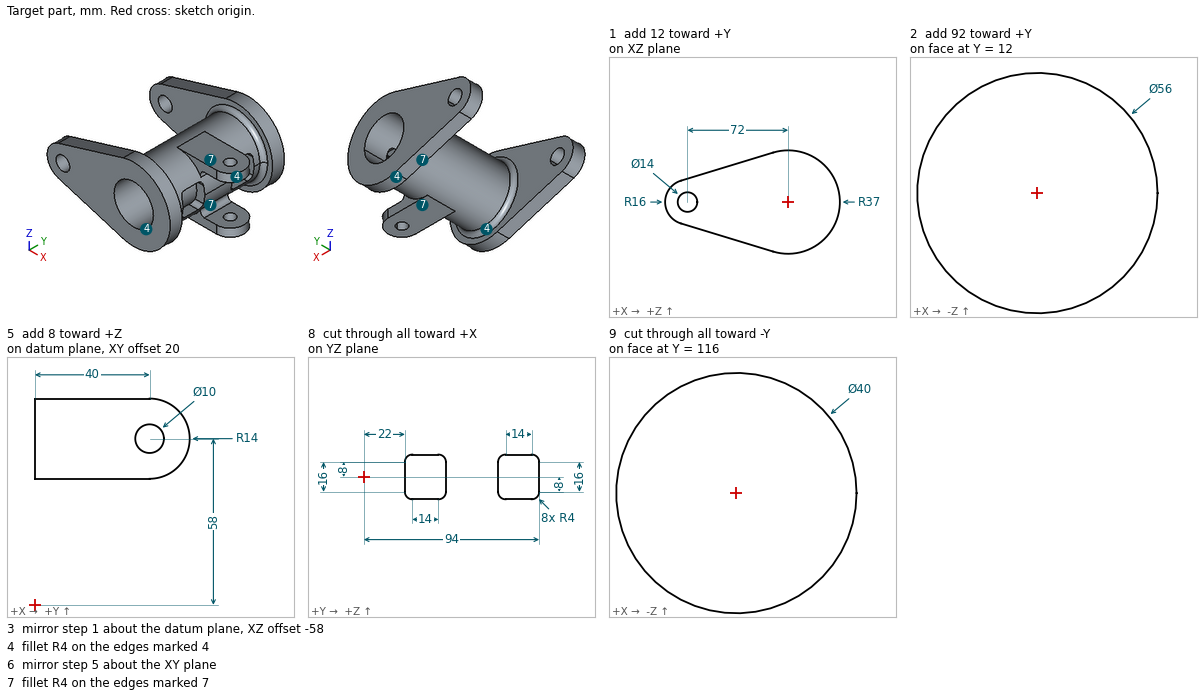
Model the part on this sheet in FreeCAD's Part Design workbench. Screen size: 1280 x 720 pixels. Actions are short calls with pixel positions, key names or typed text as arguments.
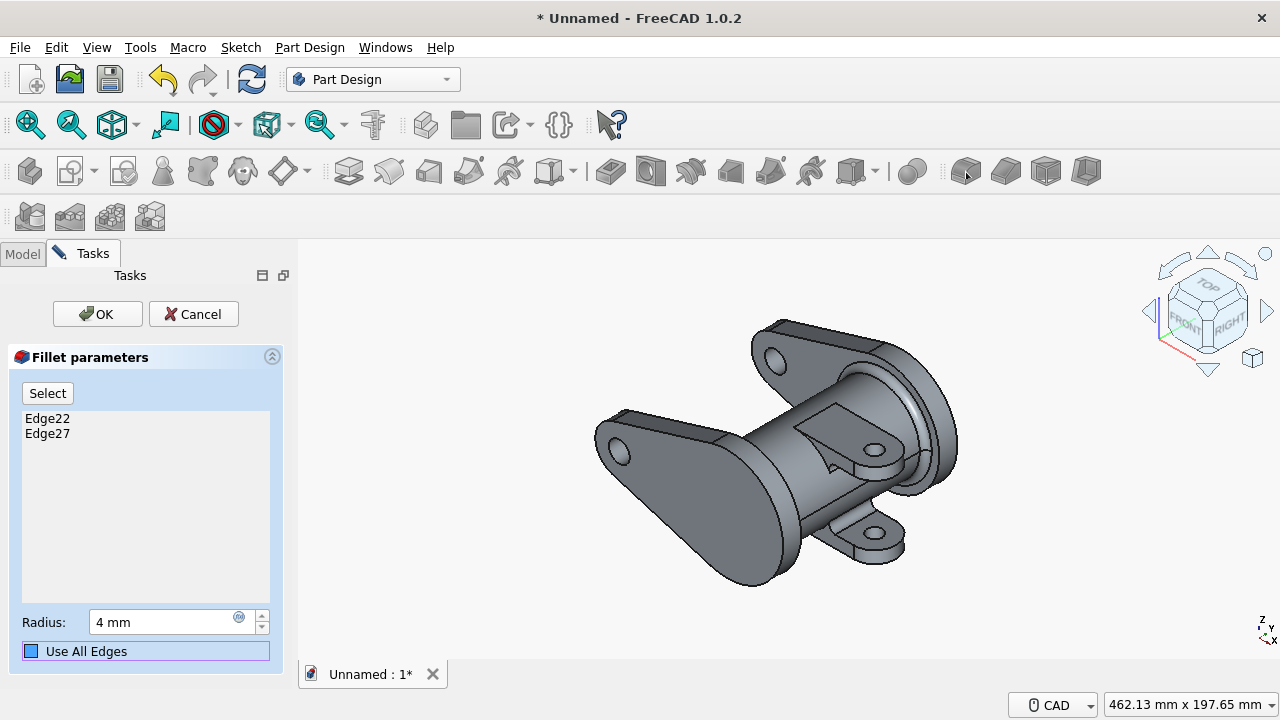
click(98, 314)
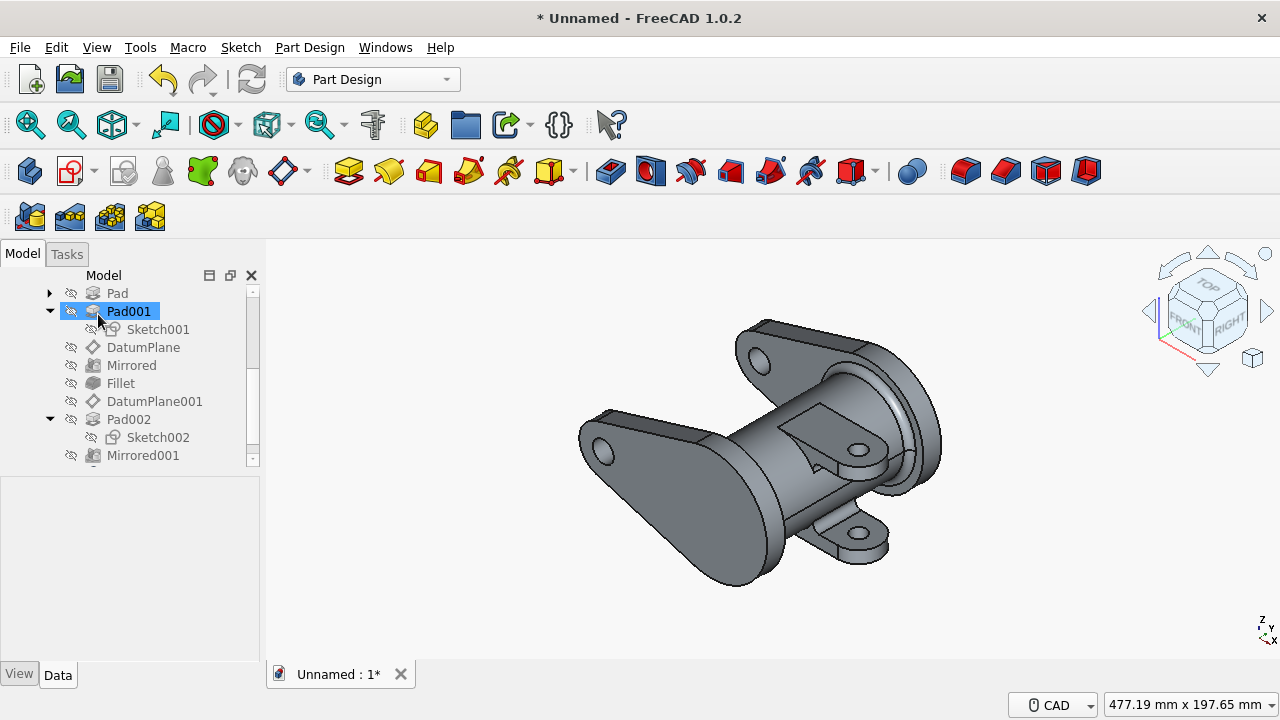
click(70, 172)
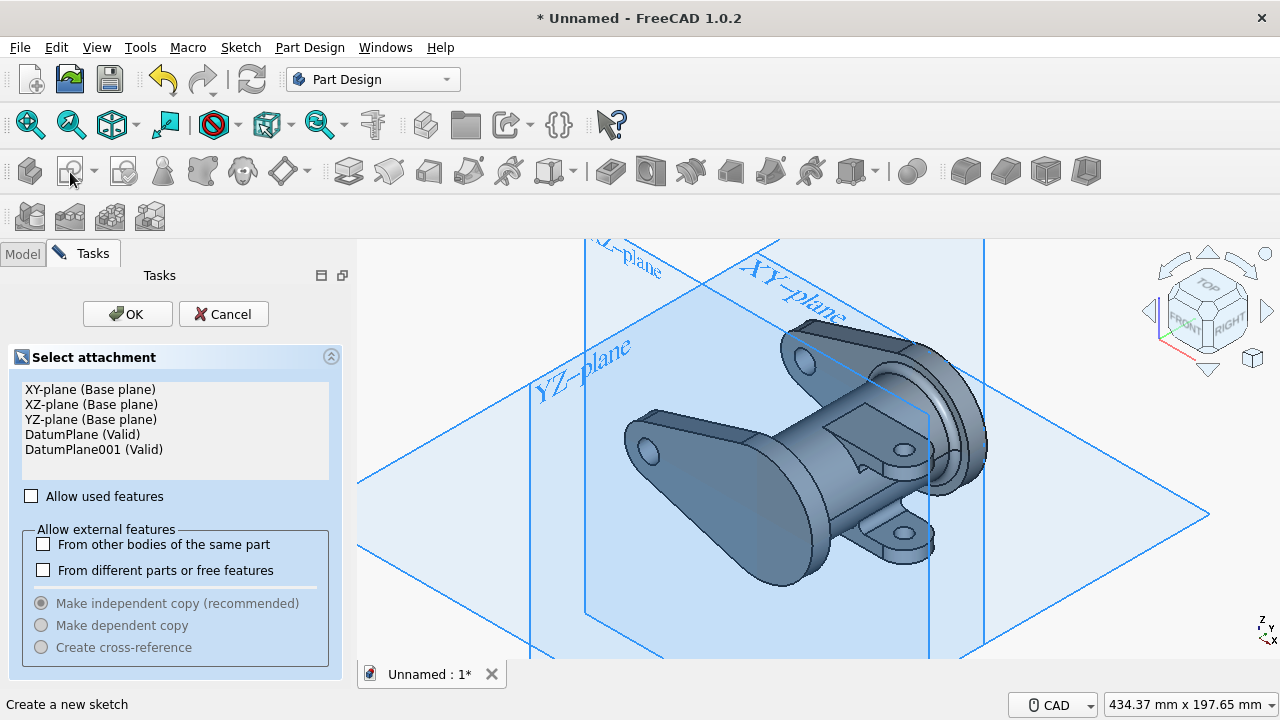
click(82, 420)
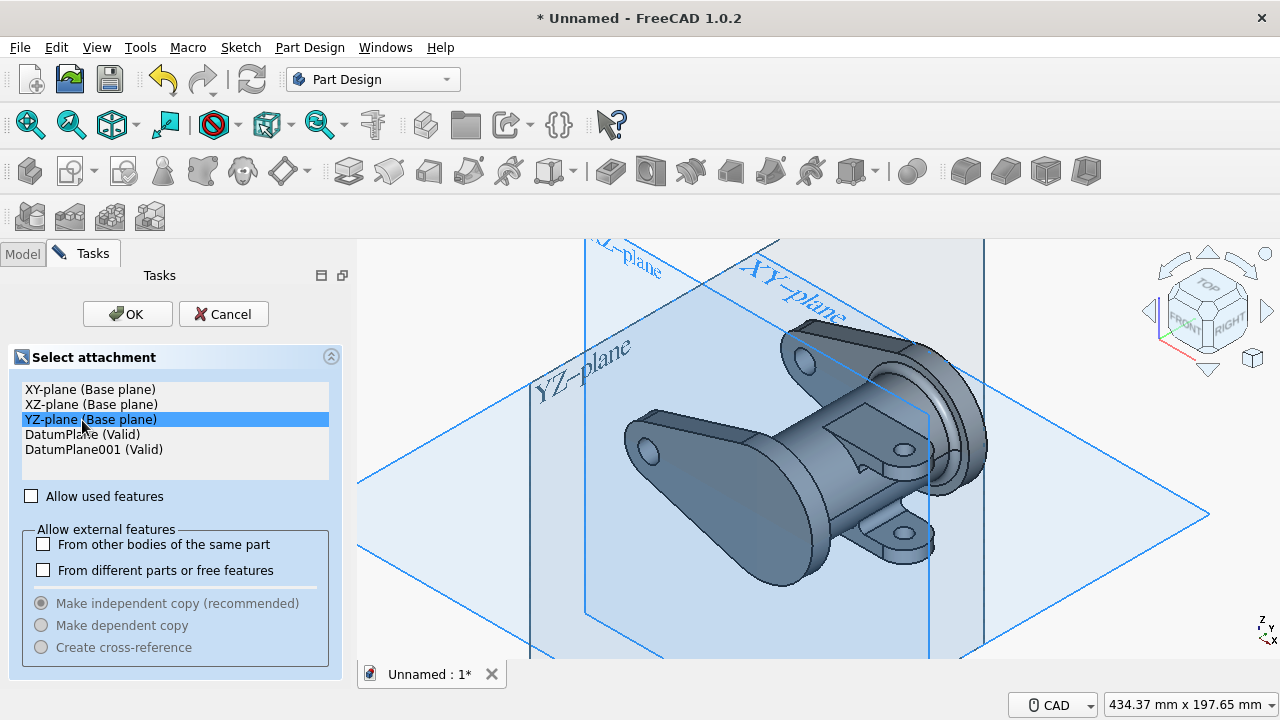
click(128, 314)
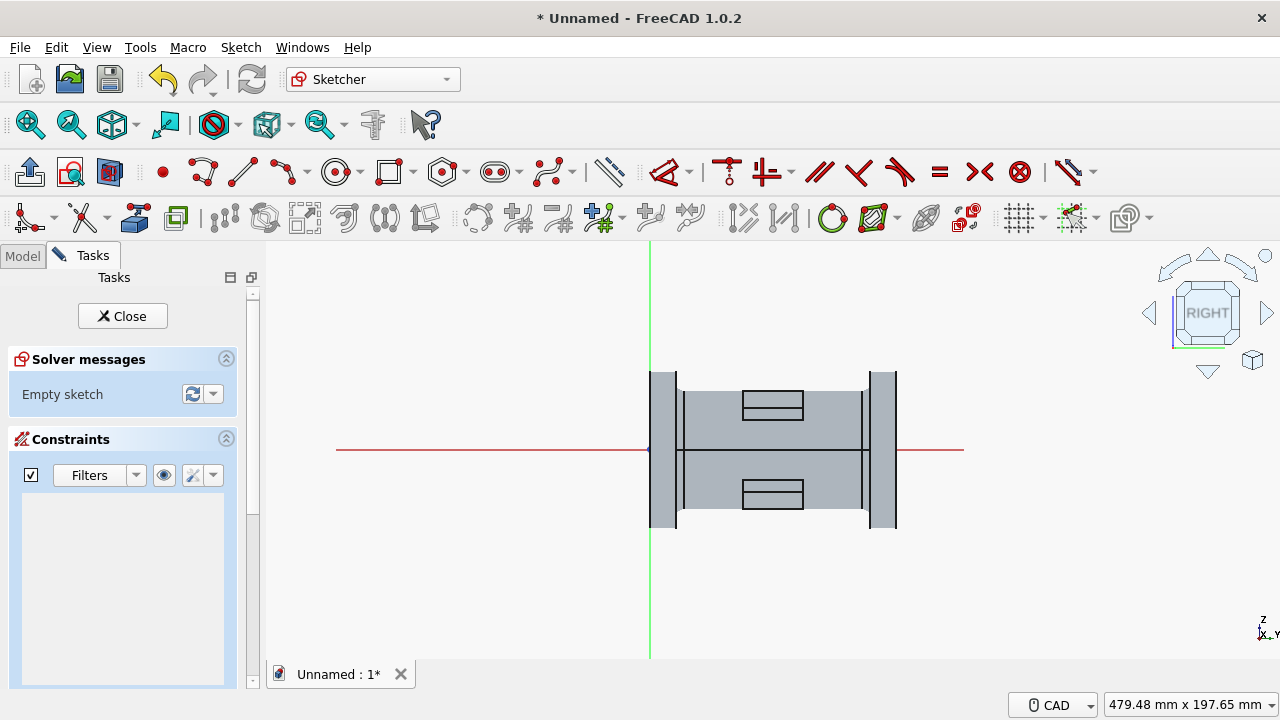
click(110, 172)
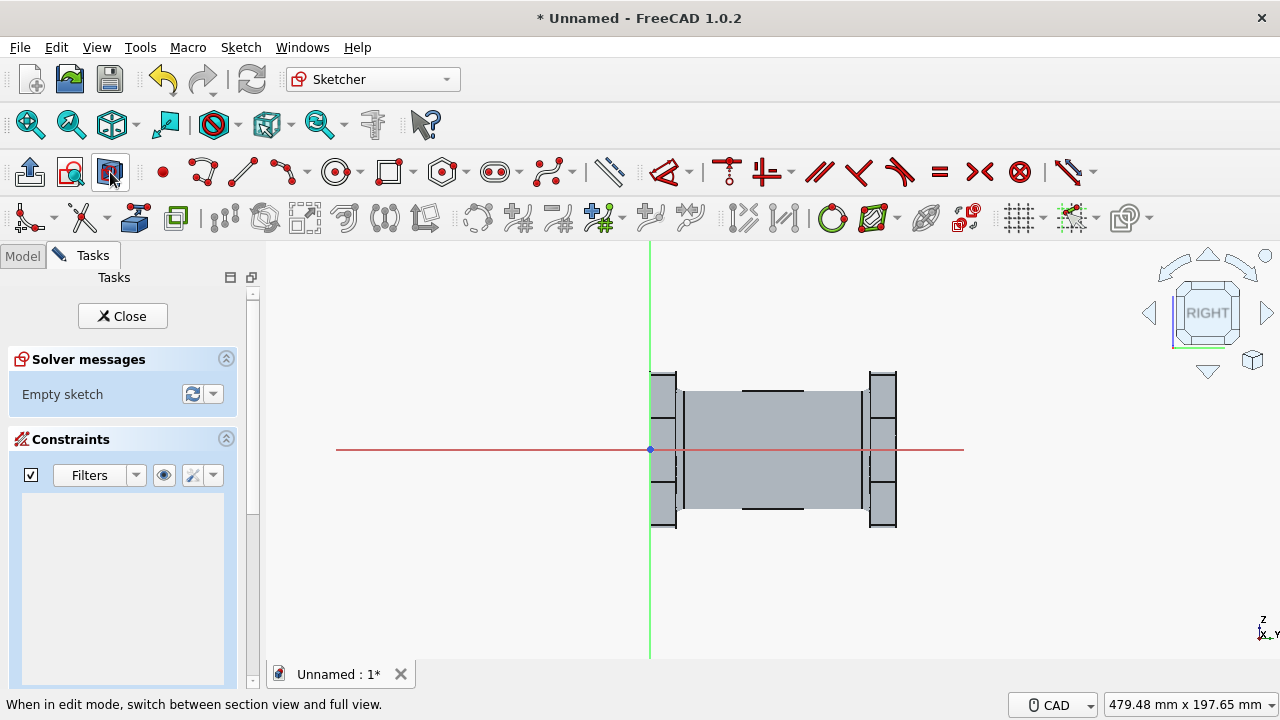
scroll(776, 450, up, 5)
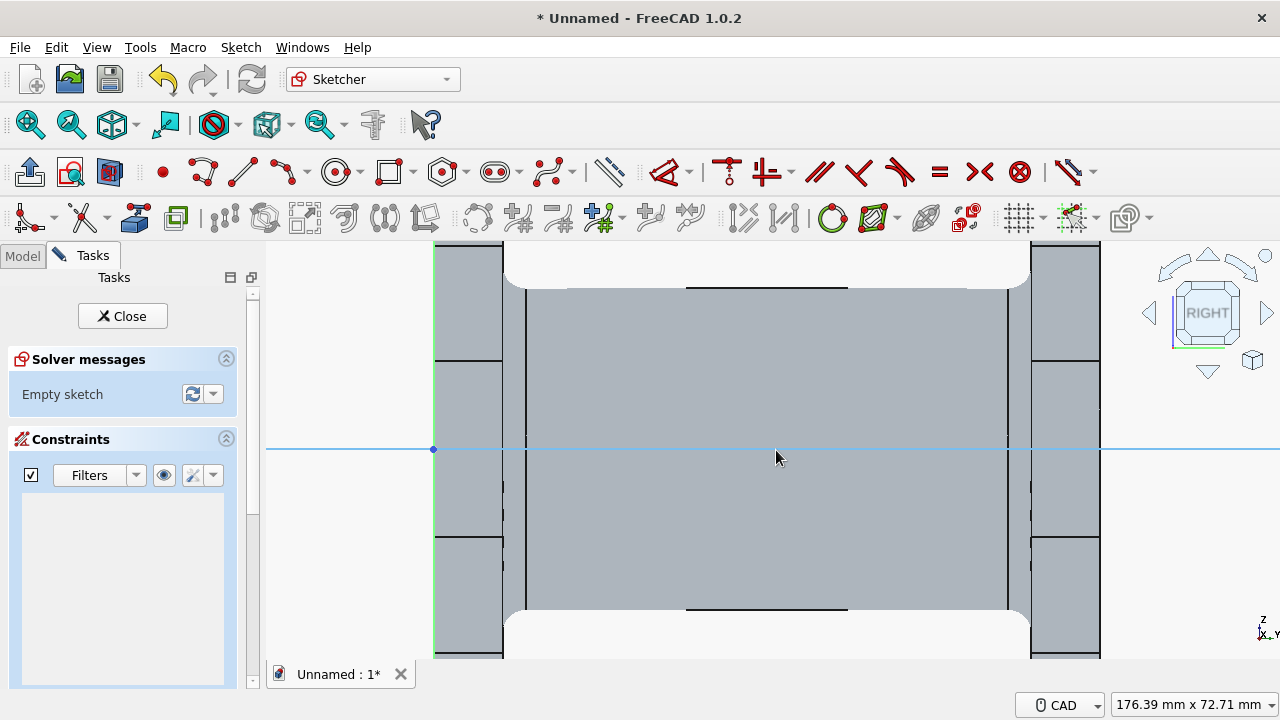
click(244, 172)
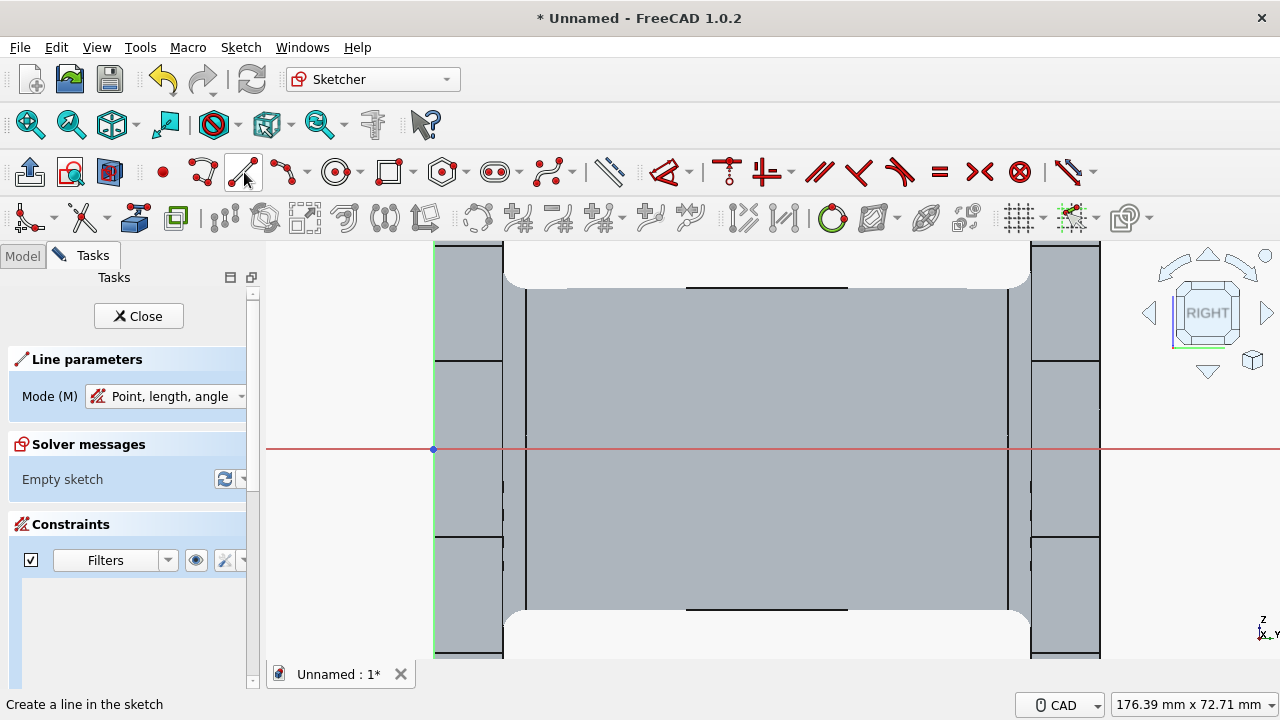
click(974, 495)
click(974, 403)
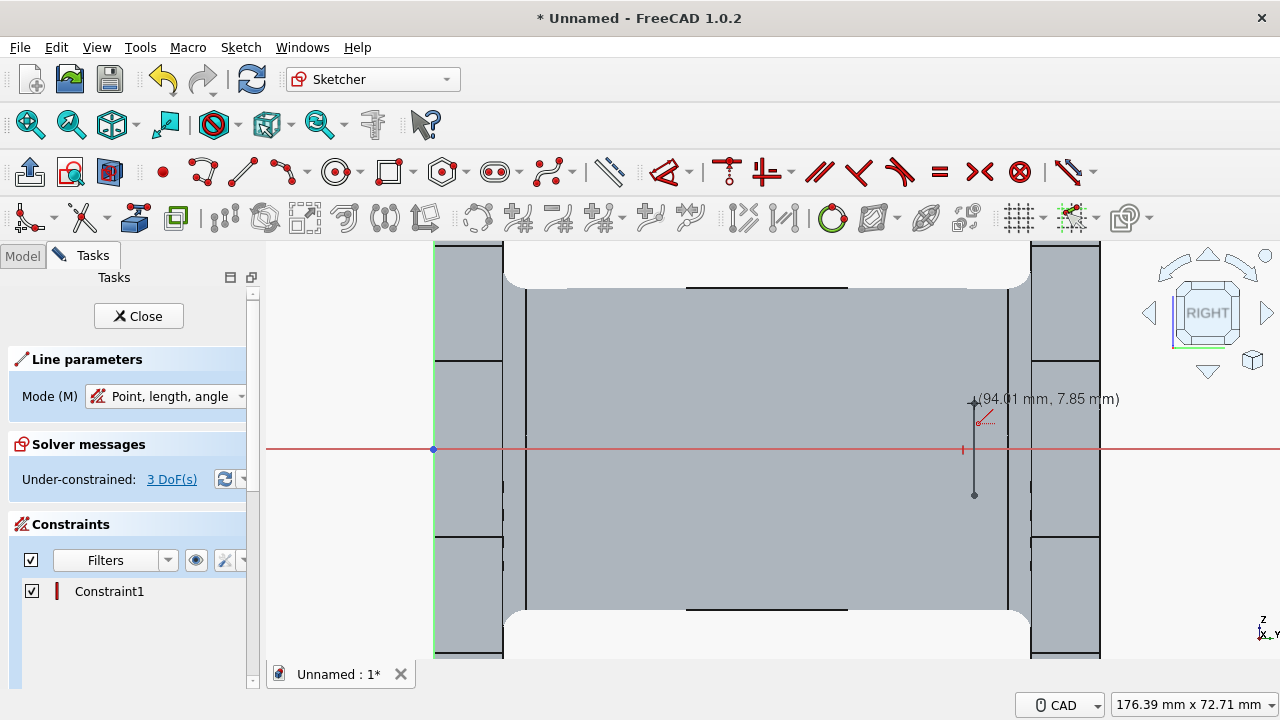
click(951, 380)
click(870, 380)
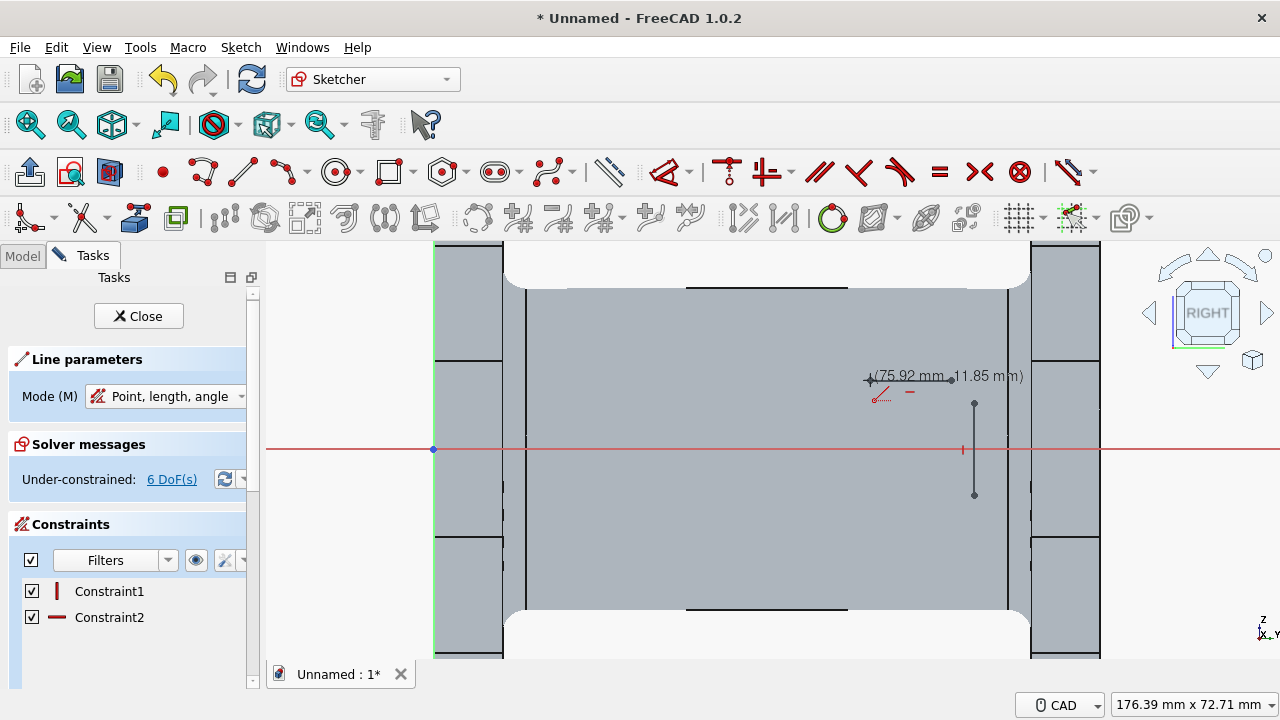
click(847, 403)
click(847, 495)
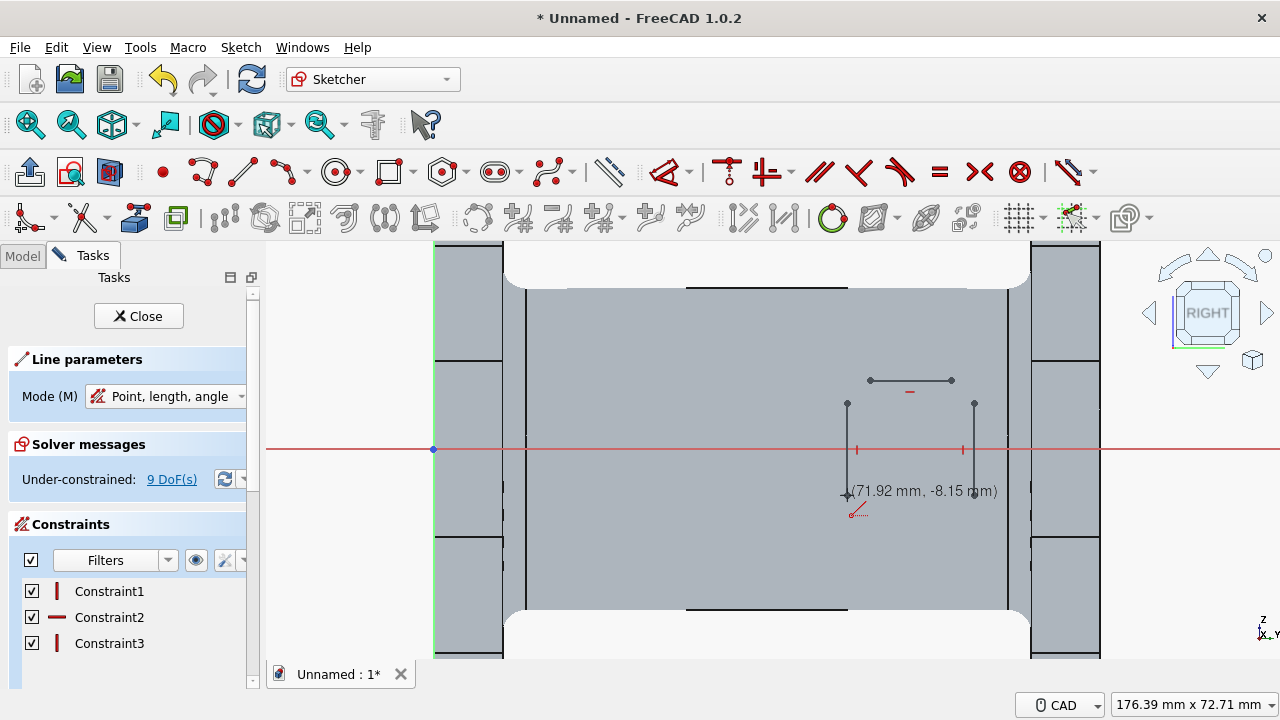
click(870, 518)
click(951, 518)